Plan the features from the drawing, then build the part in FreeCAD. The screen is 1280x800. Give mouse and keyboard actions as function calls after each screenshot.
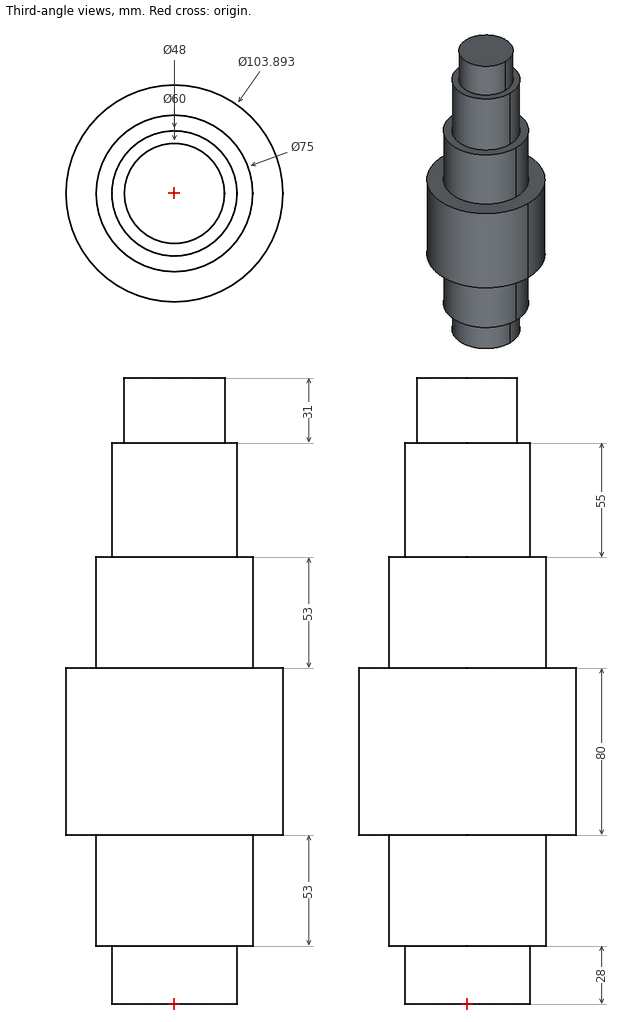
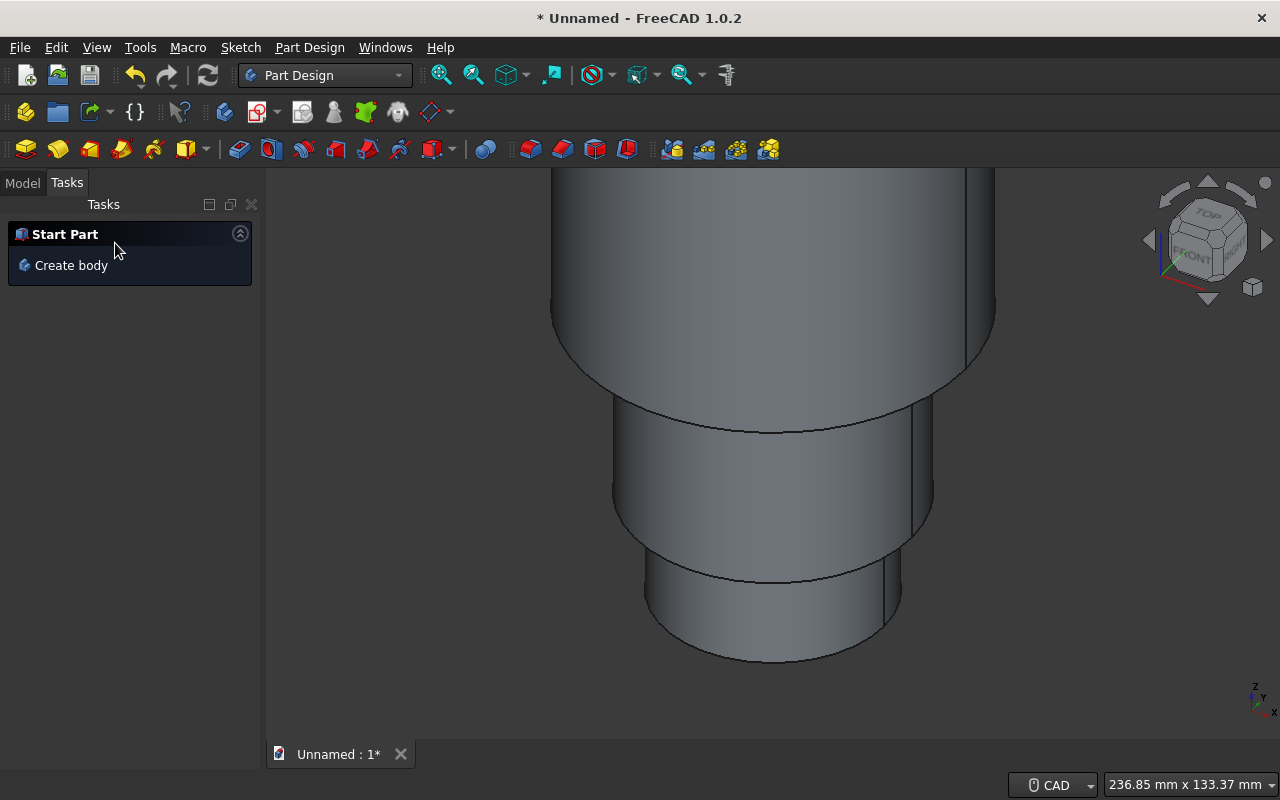
click(442, 76)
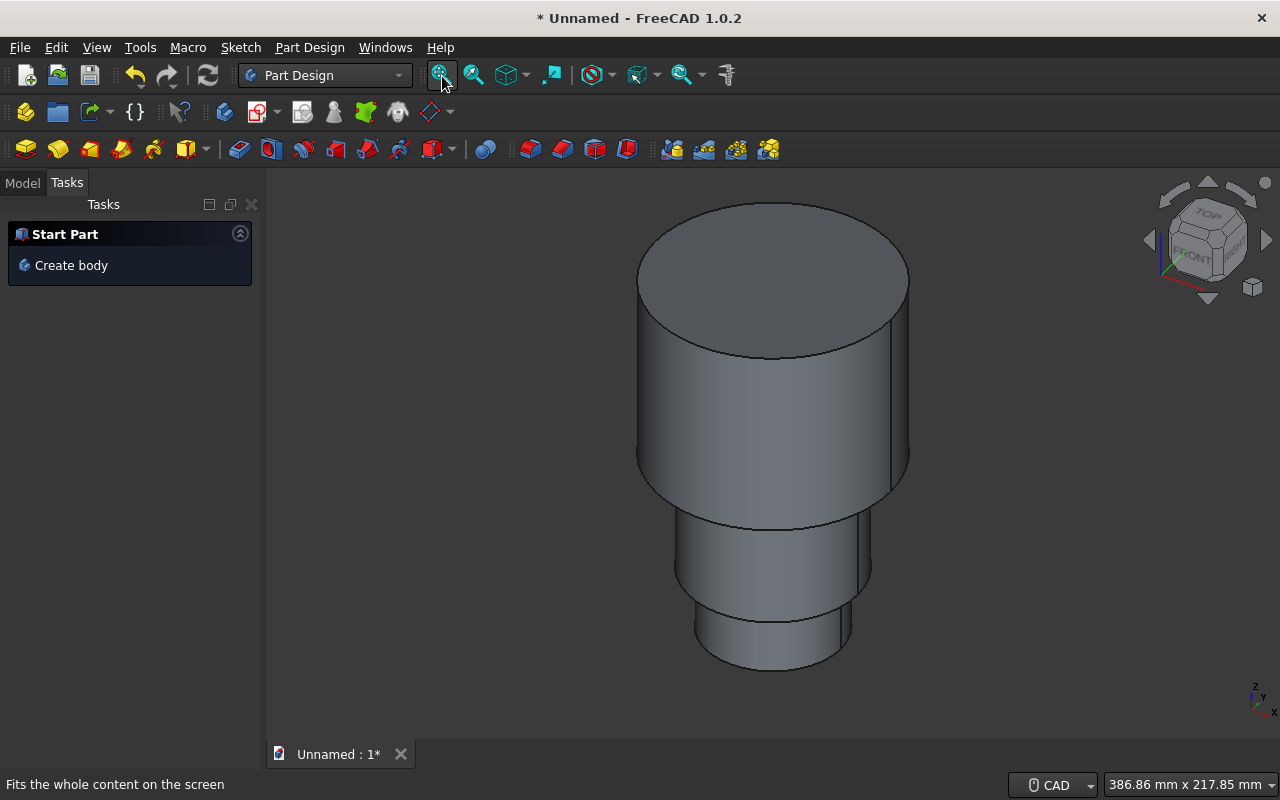
click(773, 280)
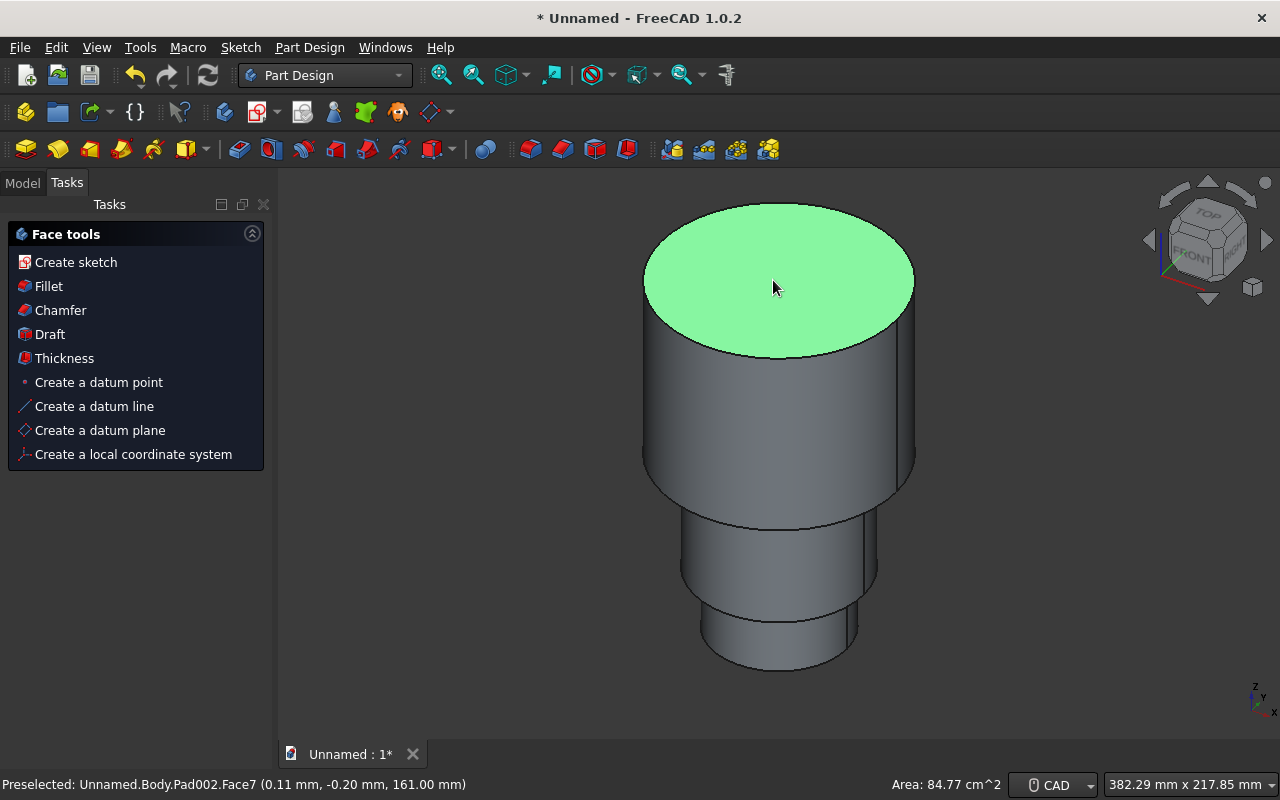
click(258, 112)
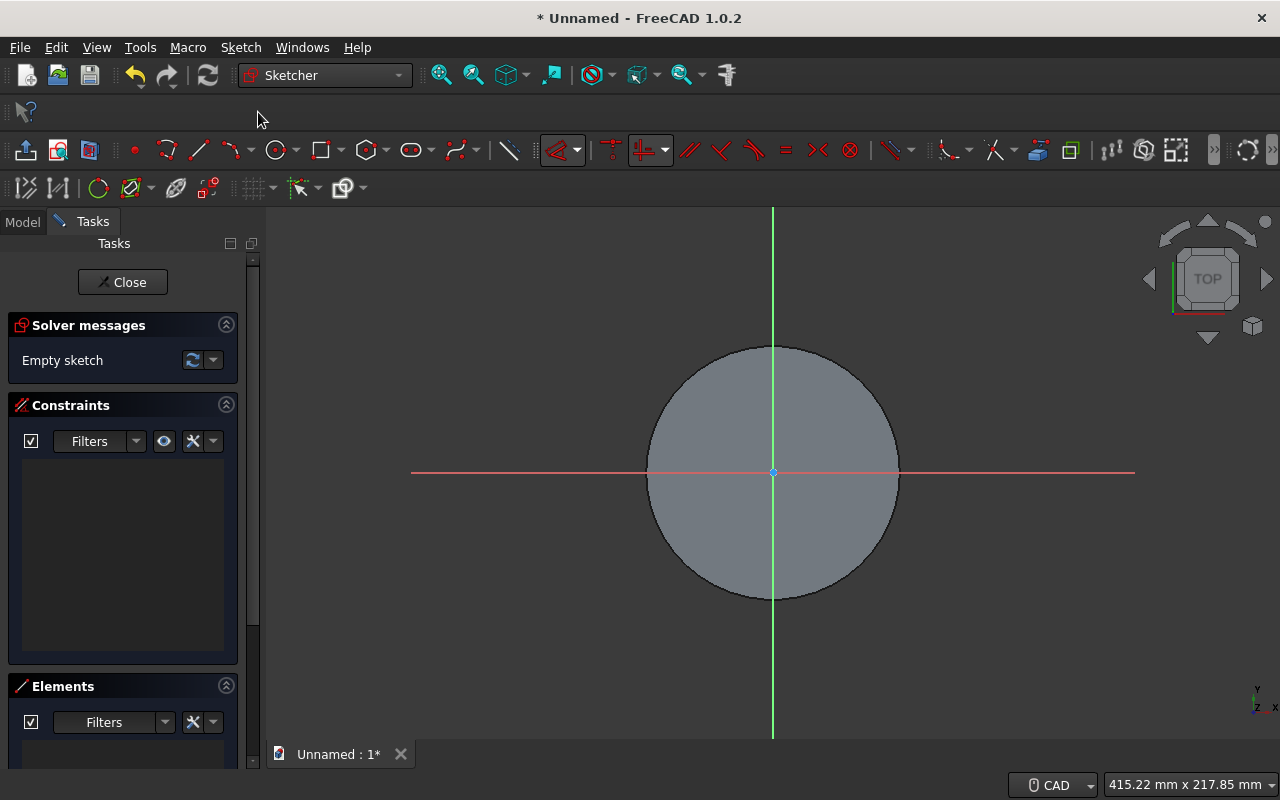
scroll(856, 473, up, 3)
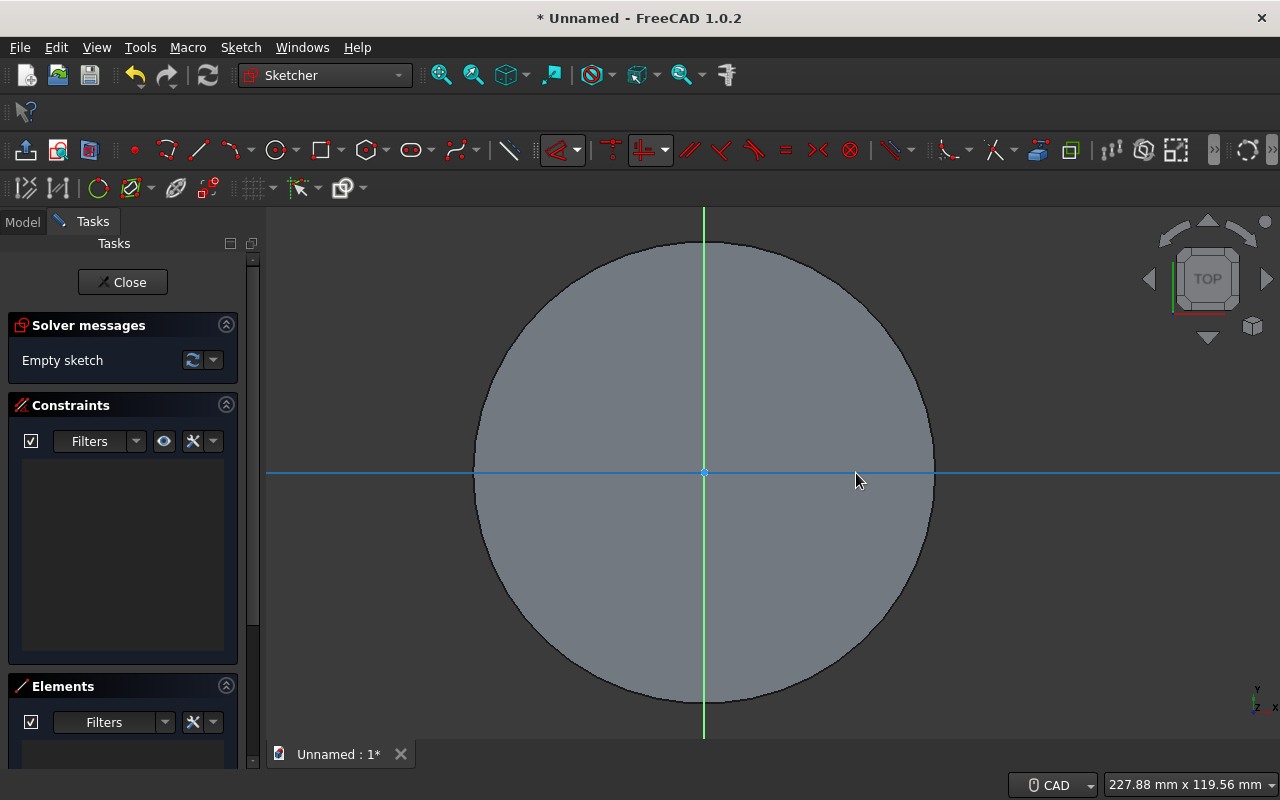
click(276, 150)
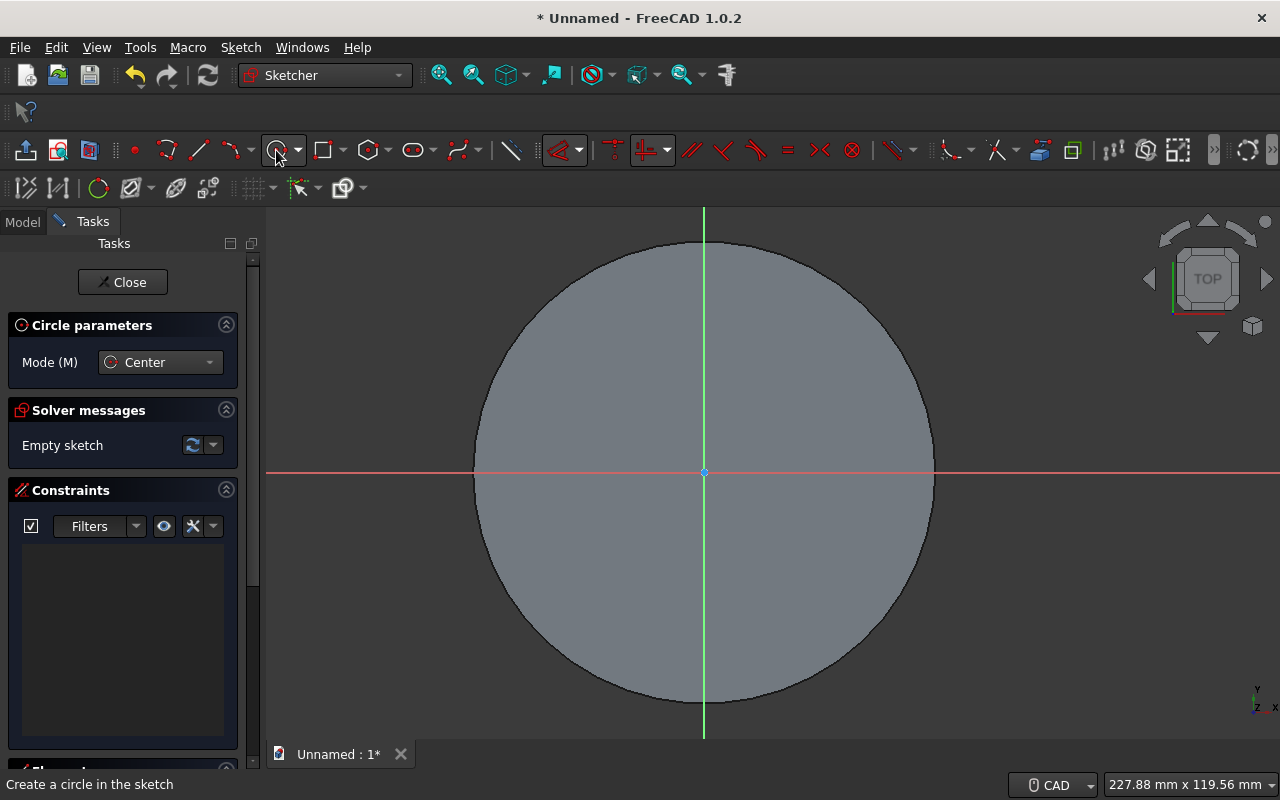
click(704, 473)
move(822, 355)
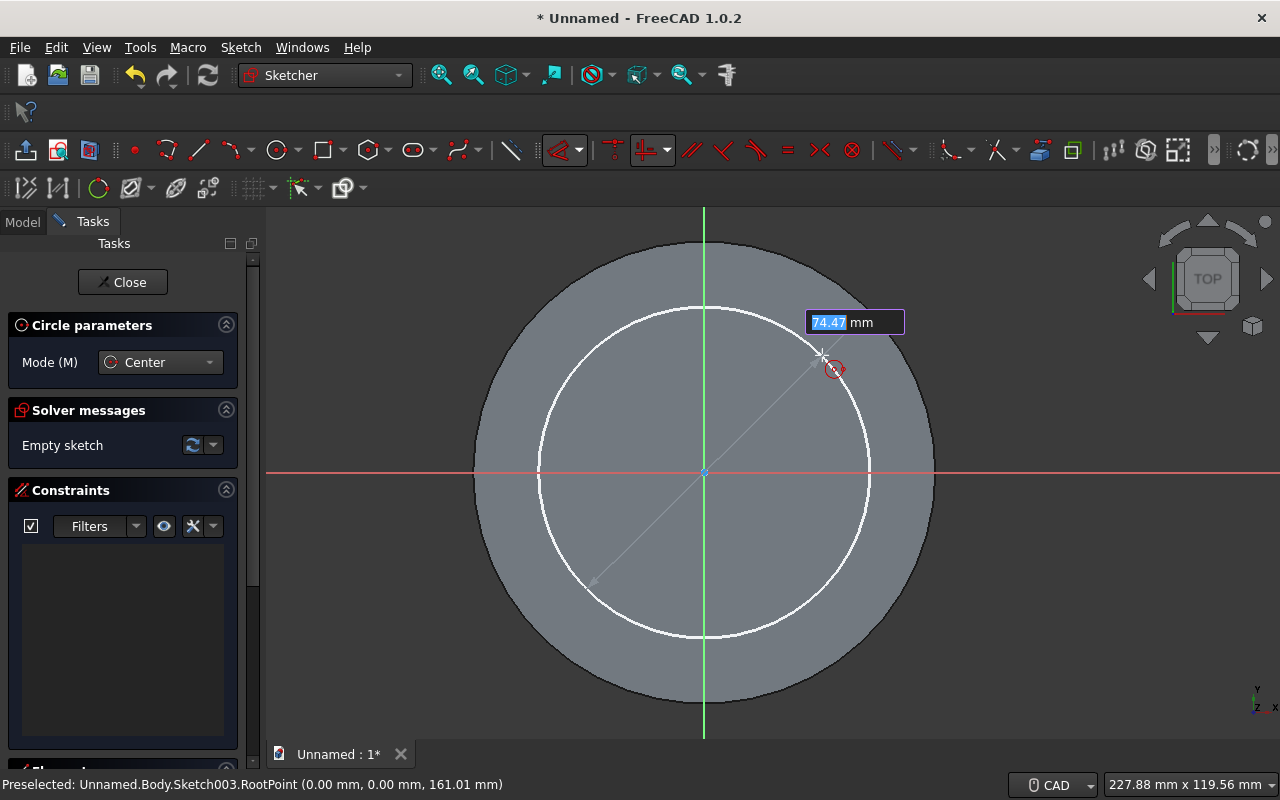
text(75)
key(Return)
key(Escape)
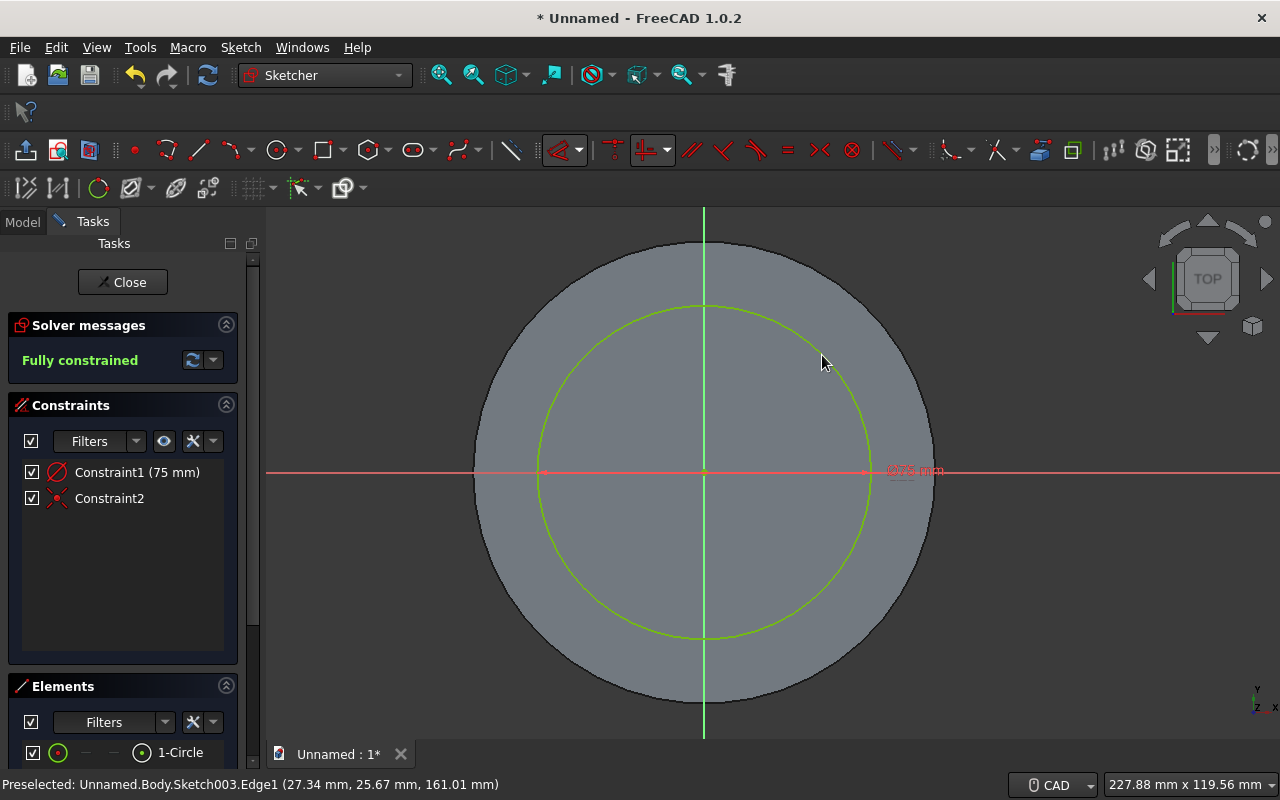
click(123, 282)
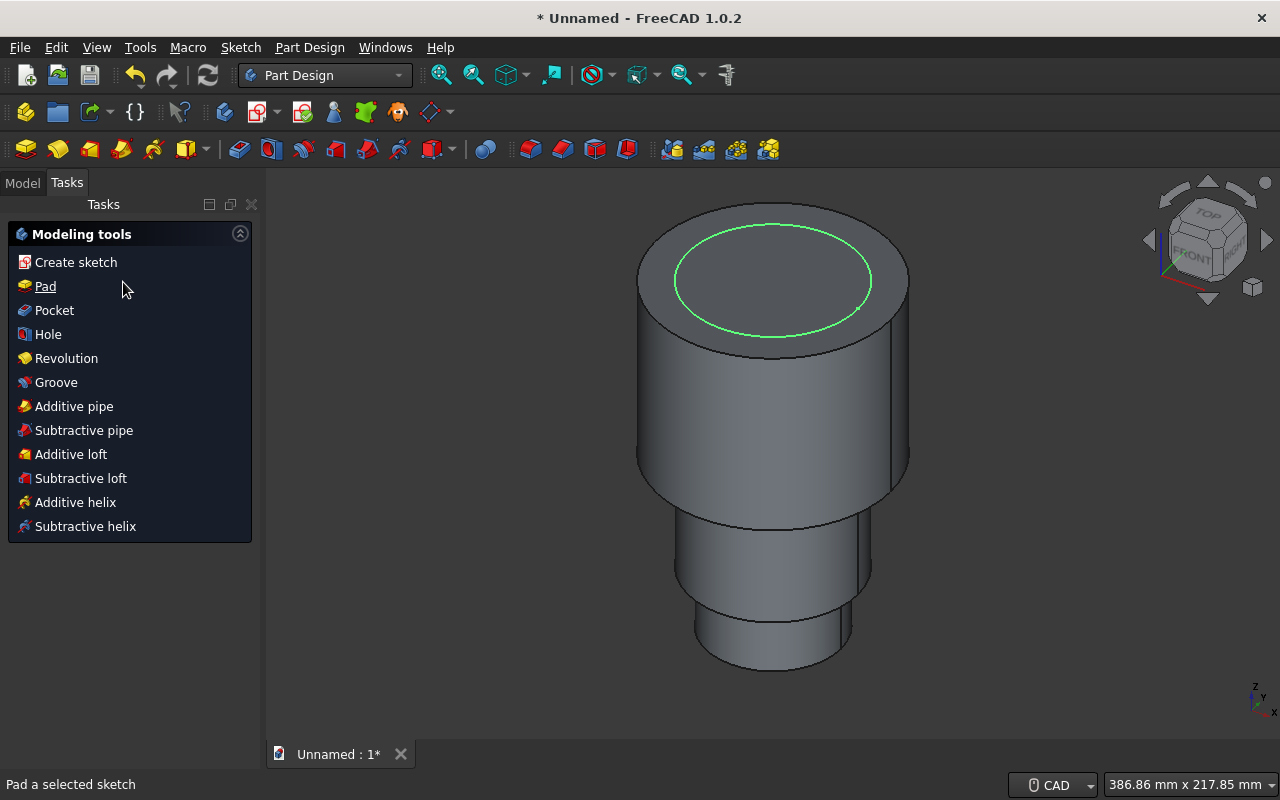
click(26, 150)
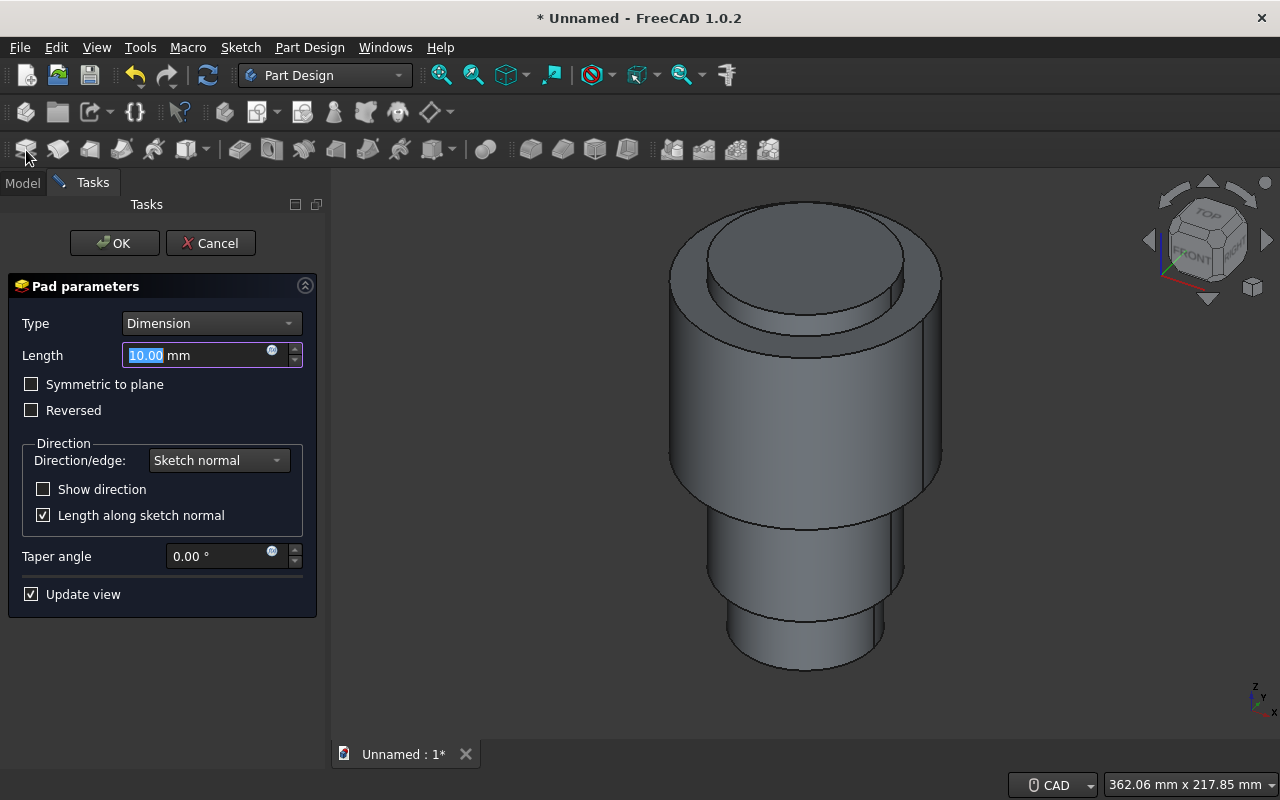
text(53)
key(Tab)